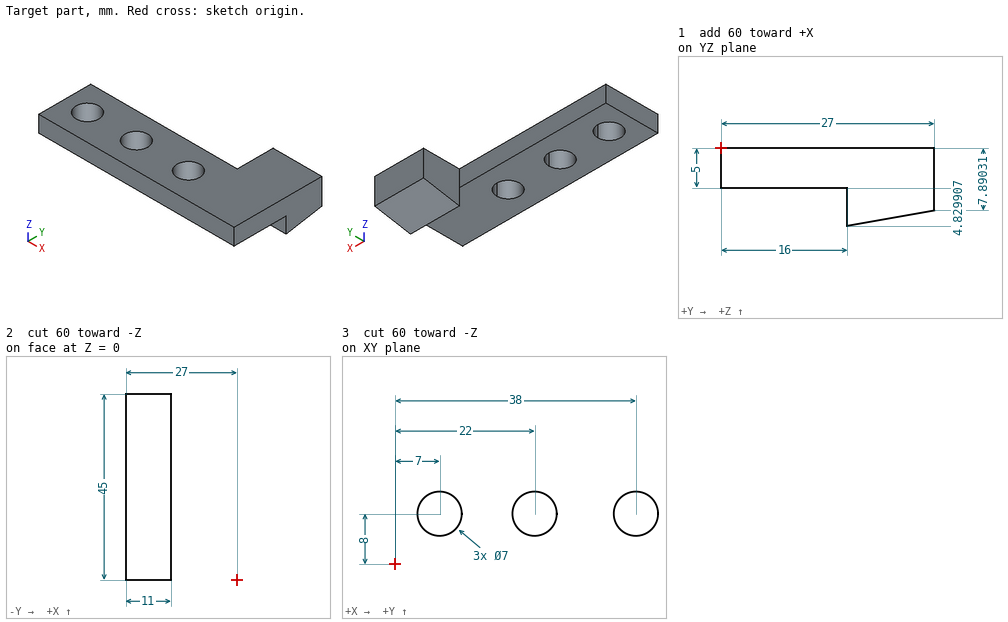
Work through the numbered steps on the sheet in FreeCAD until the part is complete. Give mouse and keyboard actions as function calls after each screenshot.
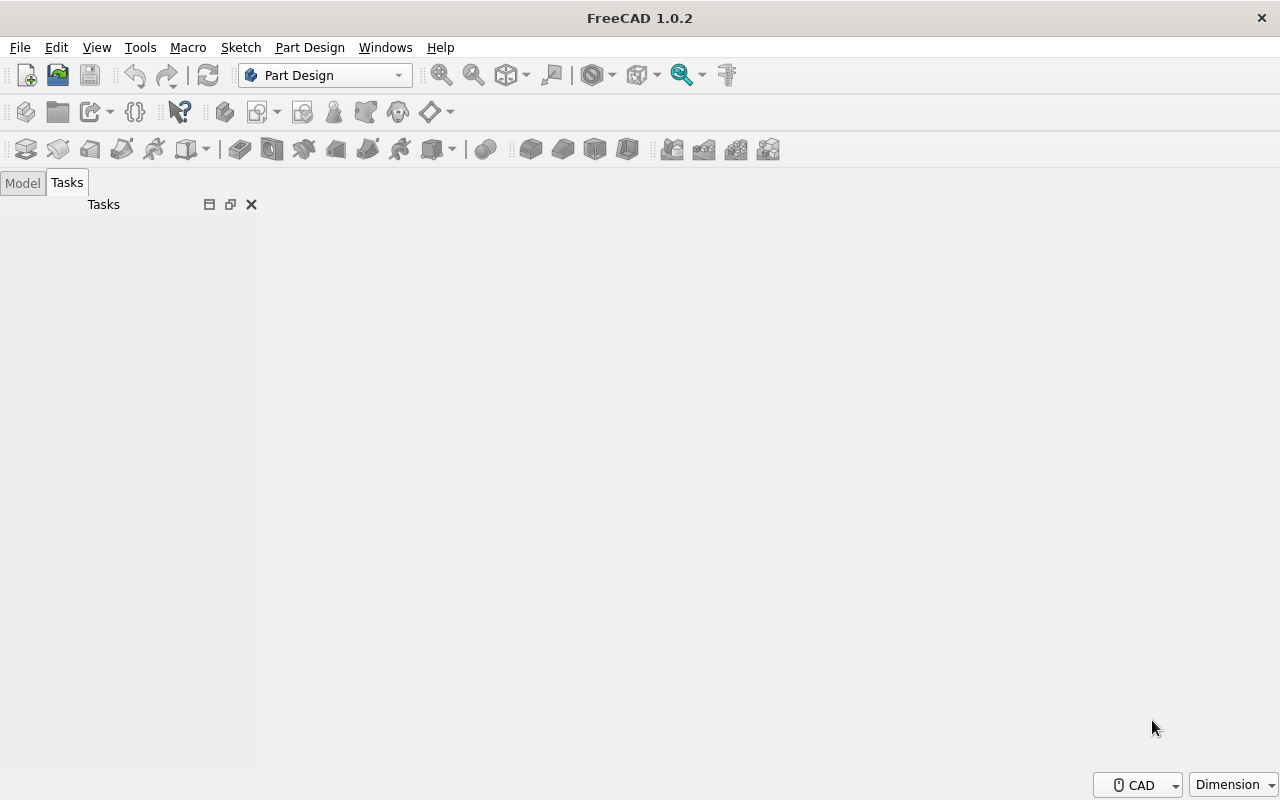
click(26, 76)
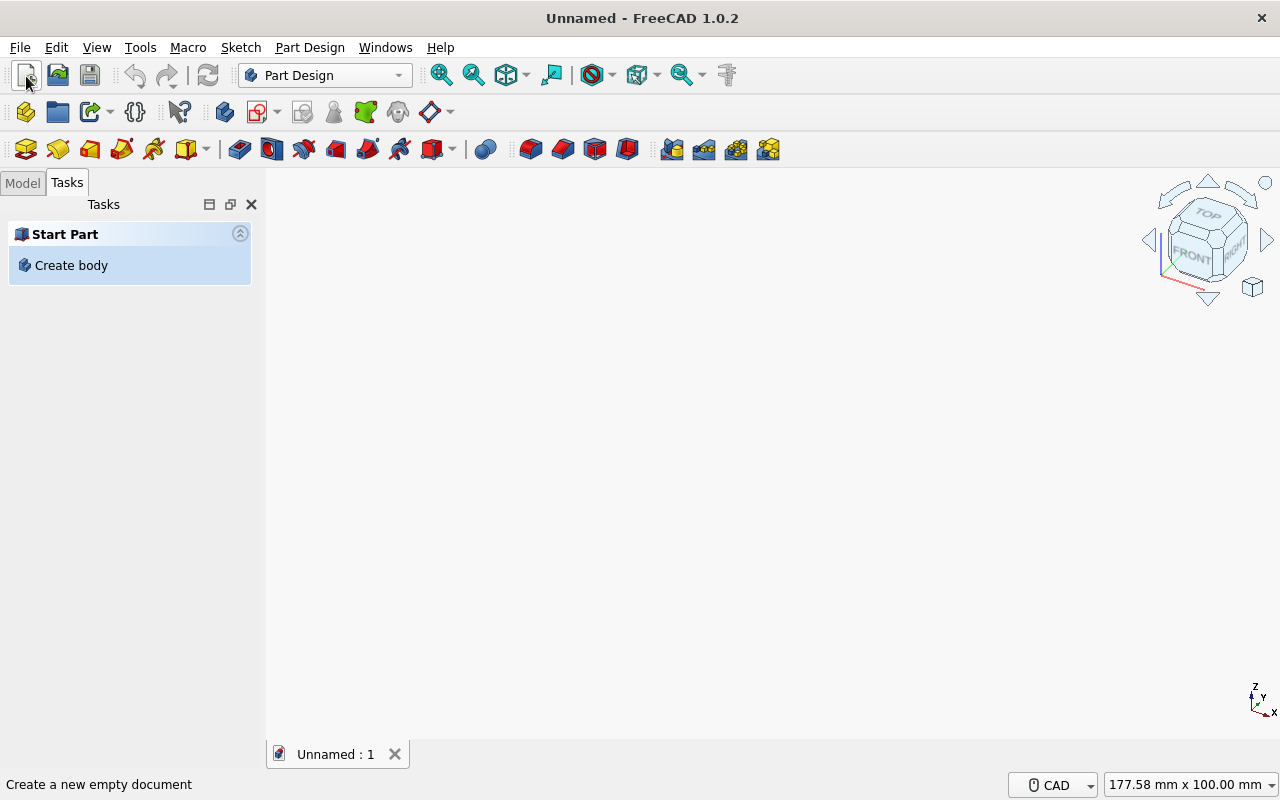
click(258, 112)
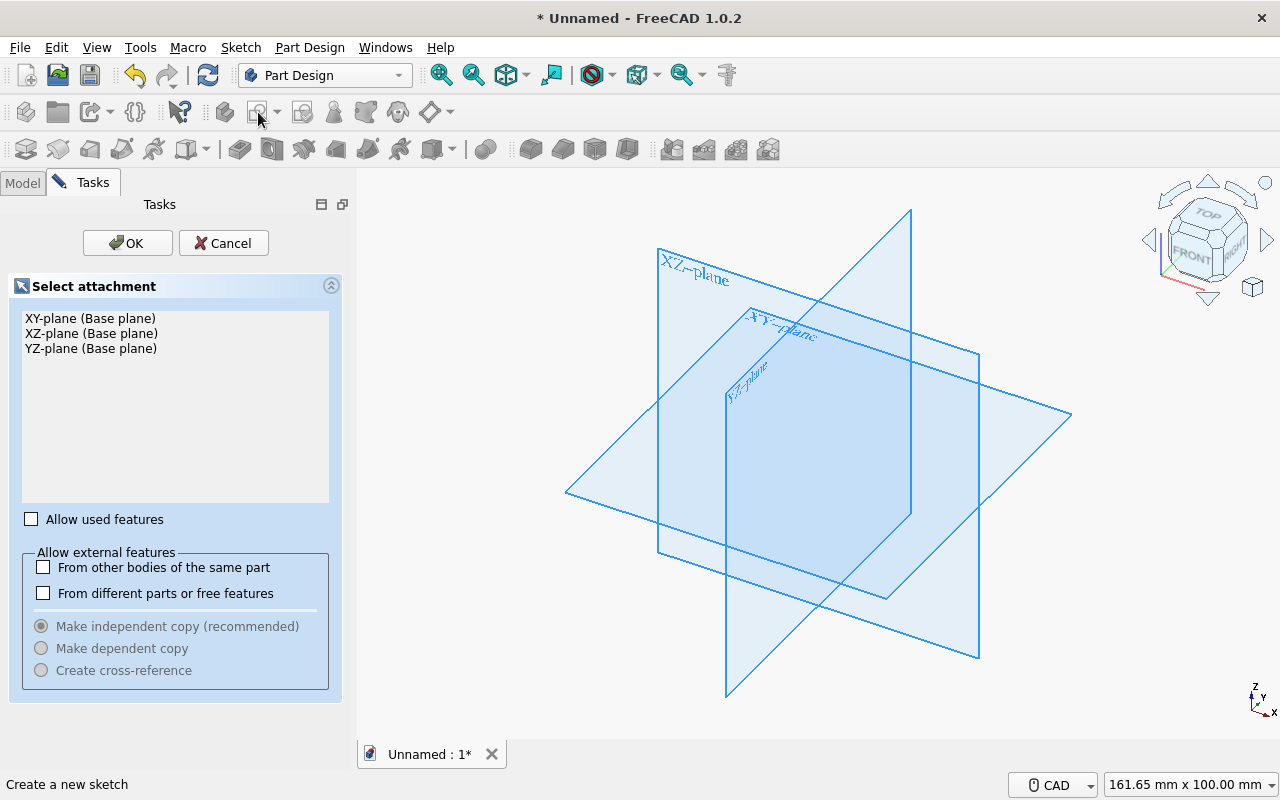
click(82, 348)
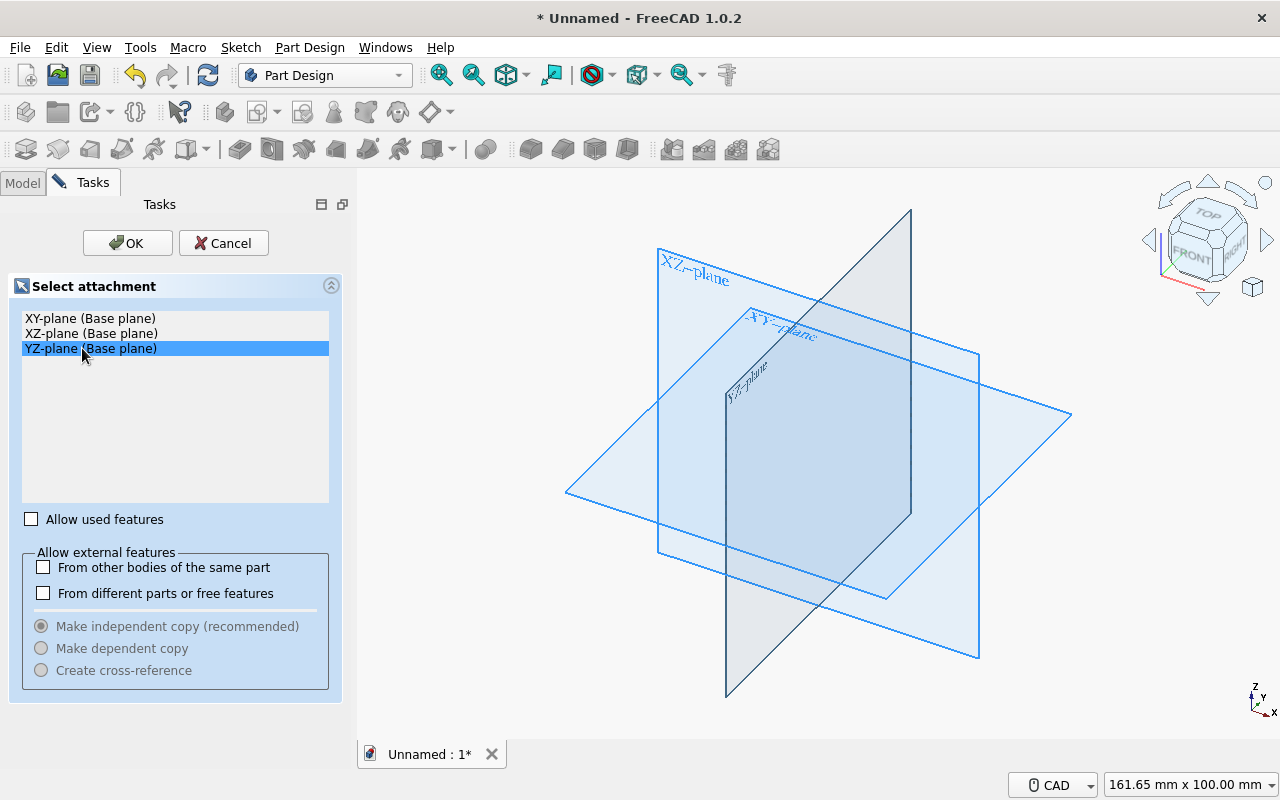
click(128, 243)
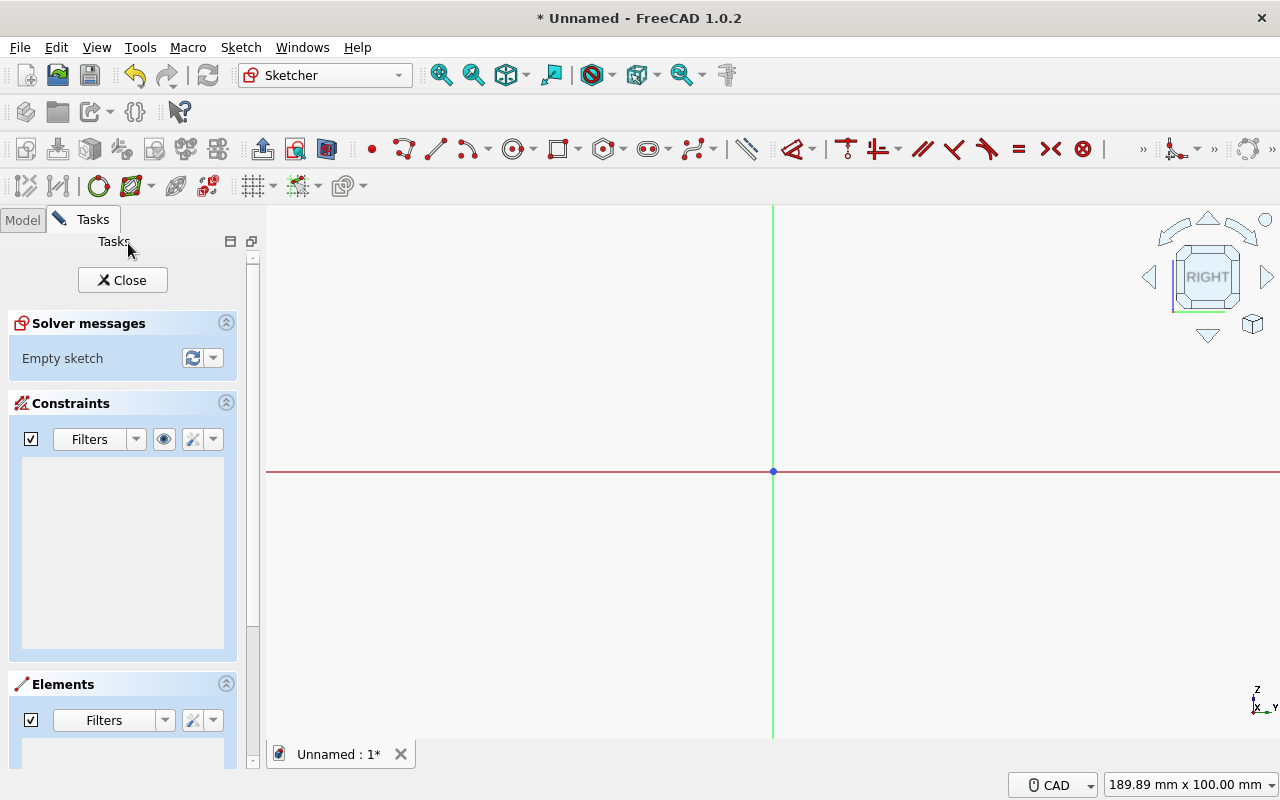
scroll(891, 507, up, 7)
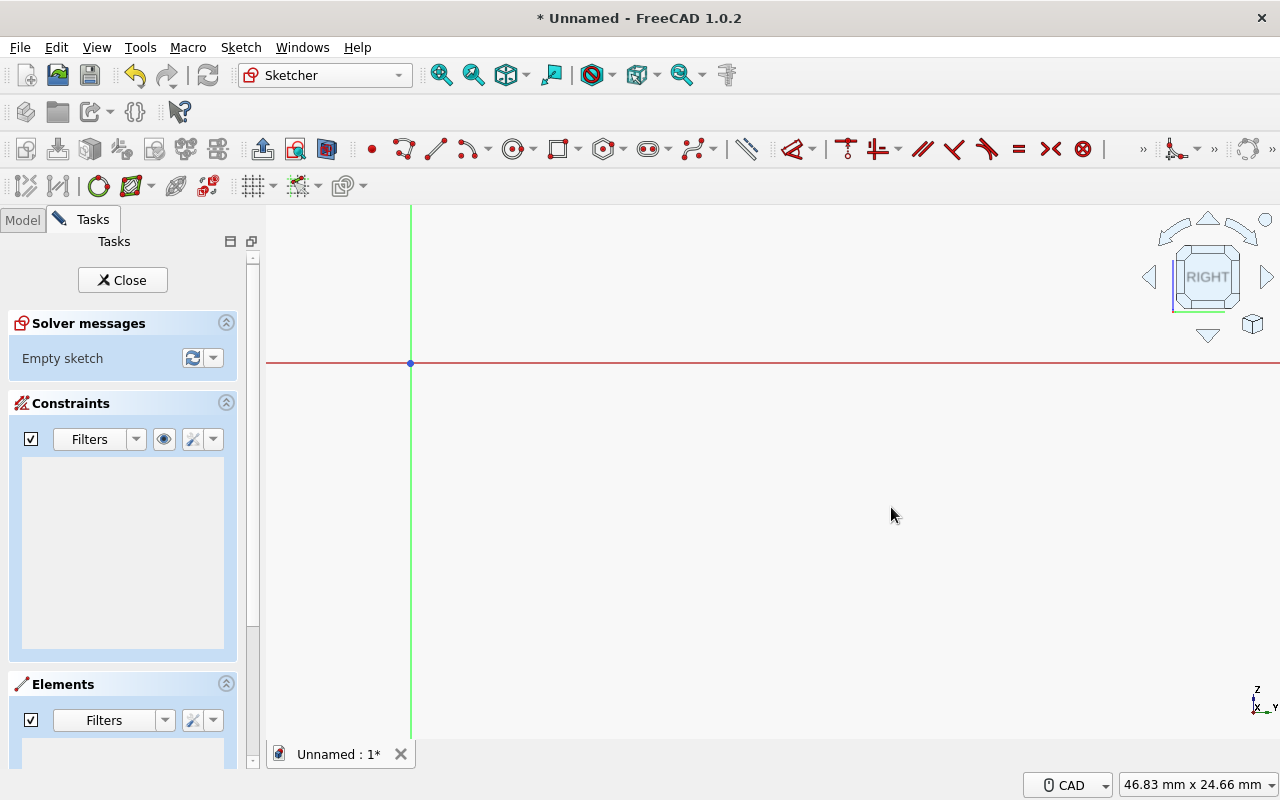
click(404, 150)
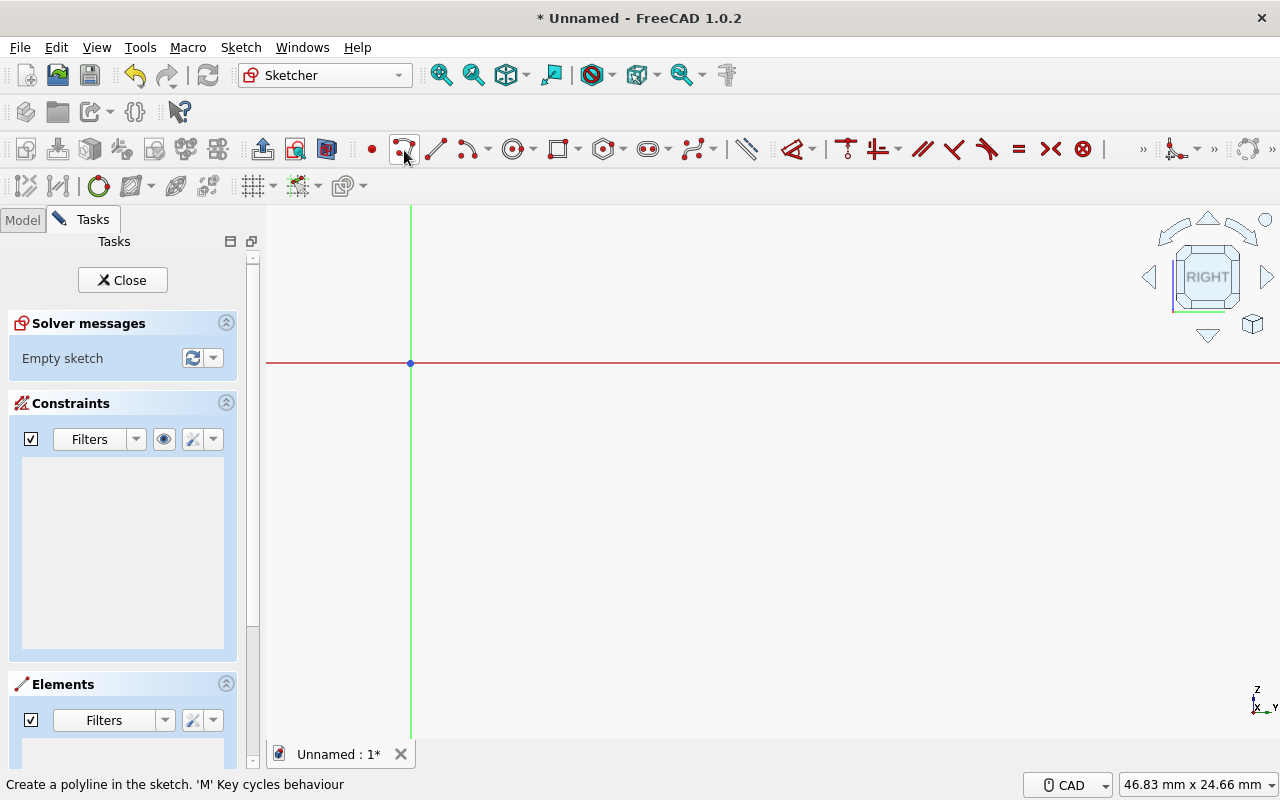
click(411, 363)
click(420, 472)
click(757, 472)
click(757, 576)
click(995, 534)
click(995, 372)
click(411, 363)
key(Escape)
key(Escape)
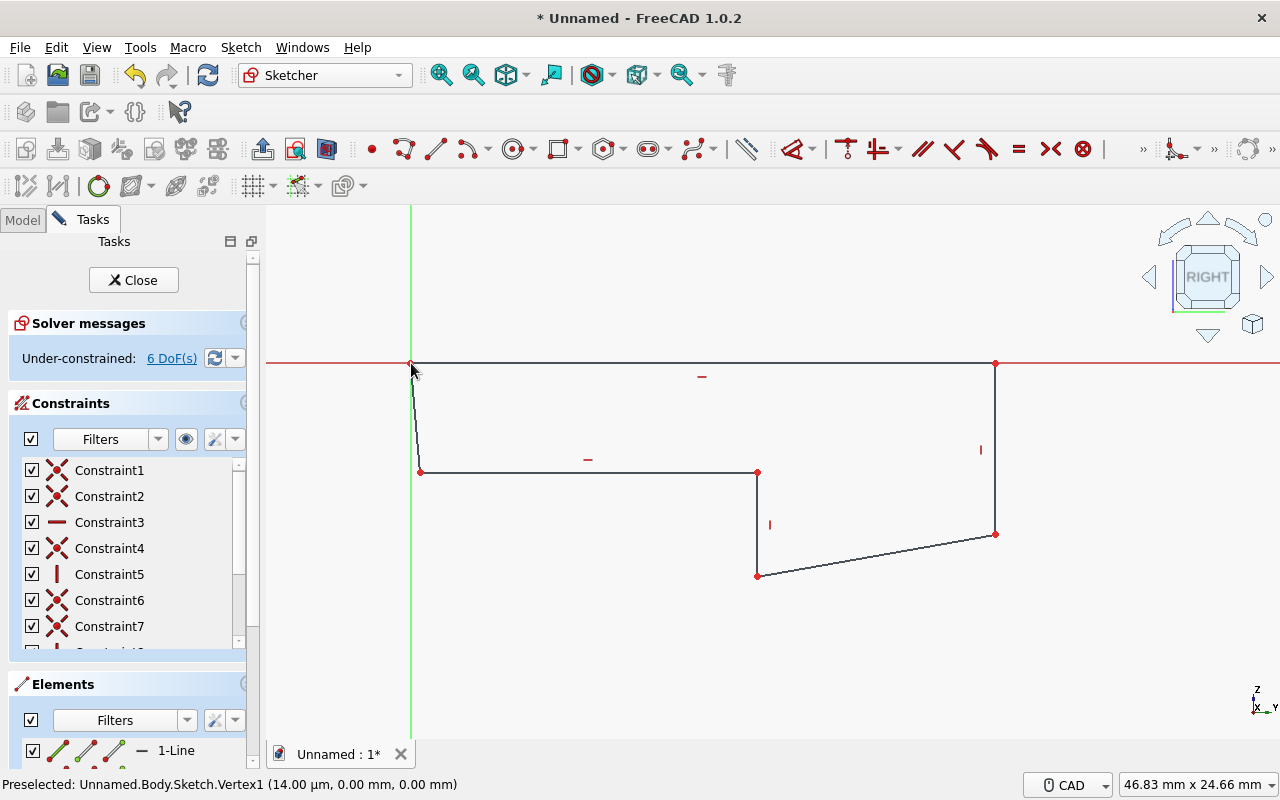
click(413, 396)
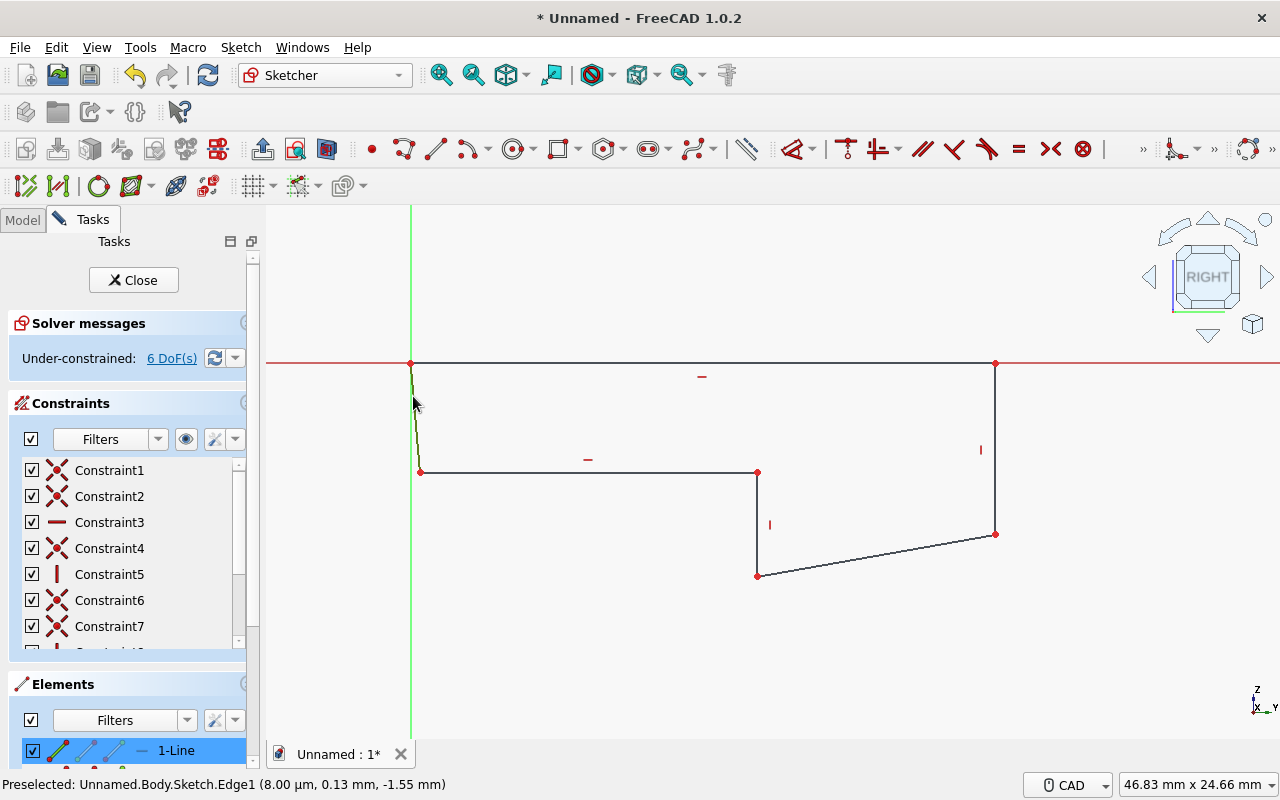
key(v)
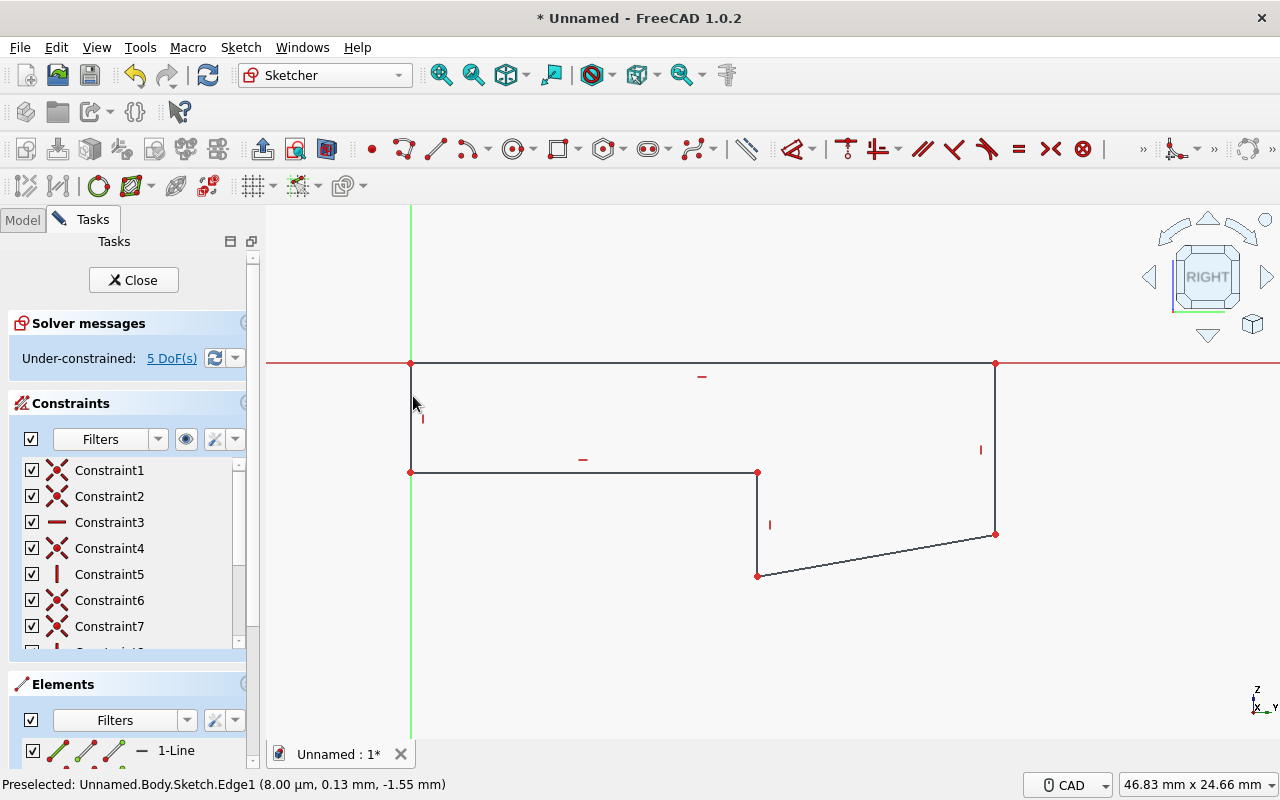
click(411, 396)